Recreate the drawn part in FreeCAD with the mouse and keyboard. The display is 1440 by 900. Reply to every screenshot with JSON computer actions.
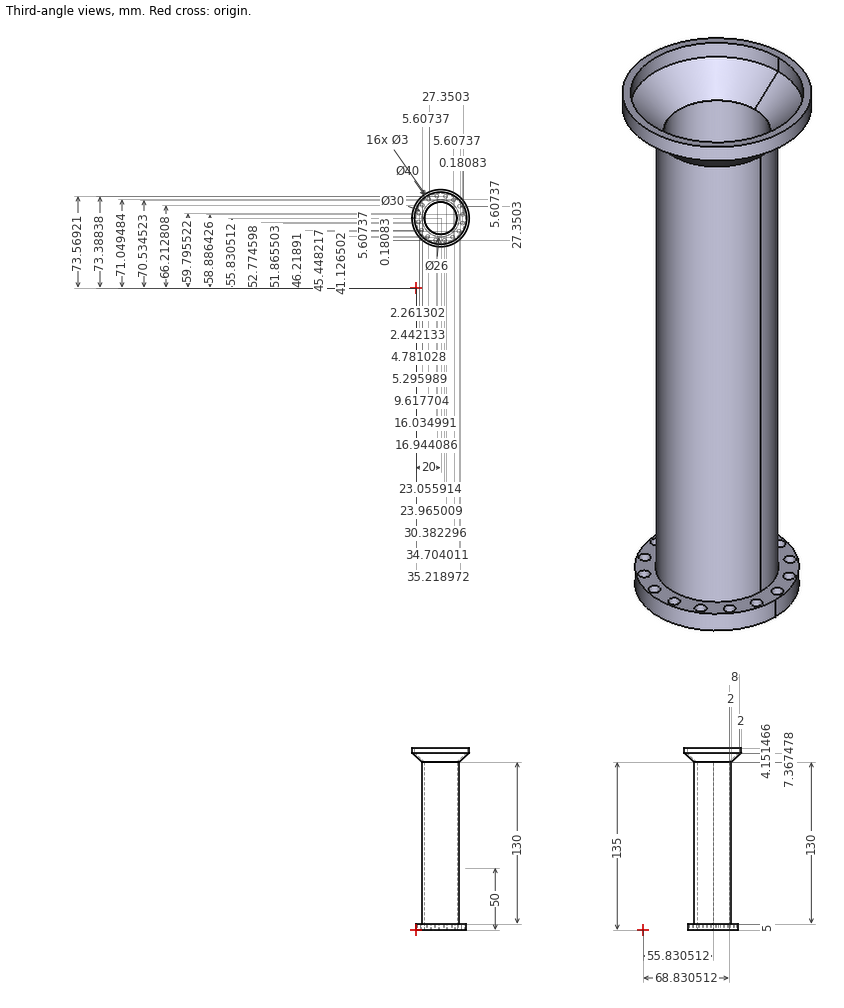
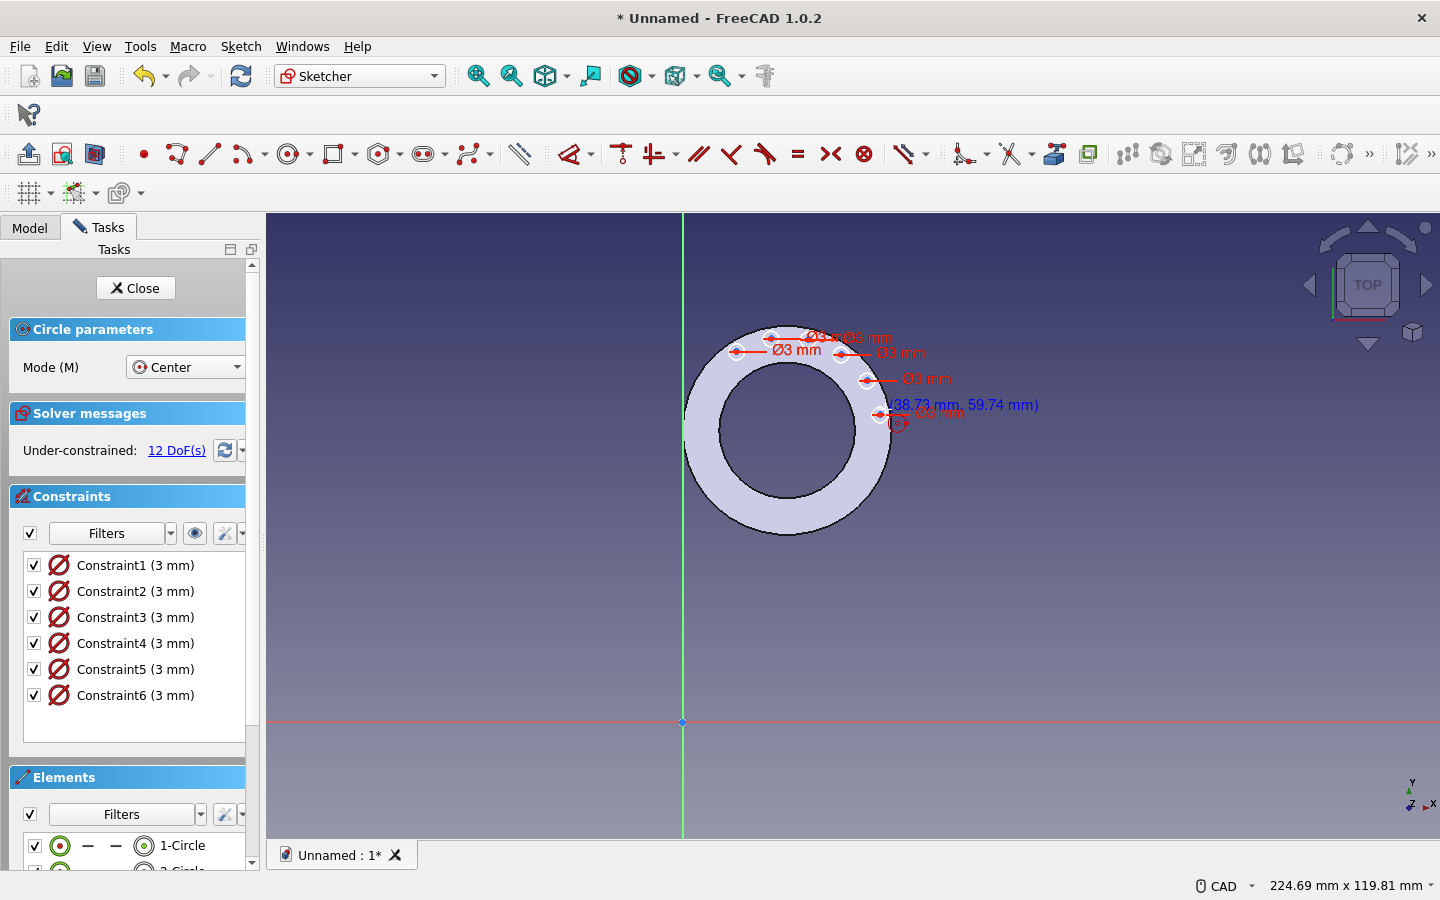
{"action": "scroll", "coordinate": [879, 451], "scroll_direction": "up", "scroll_amount": 6}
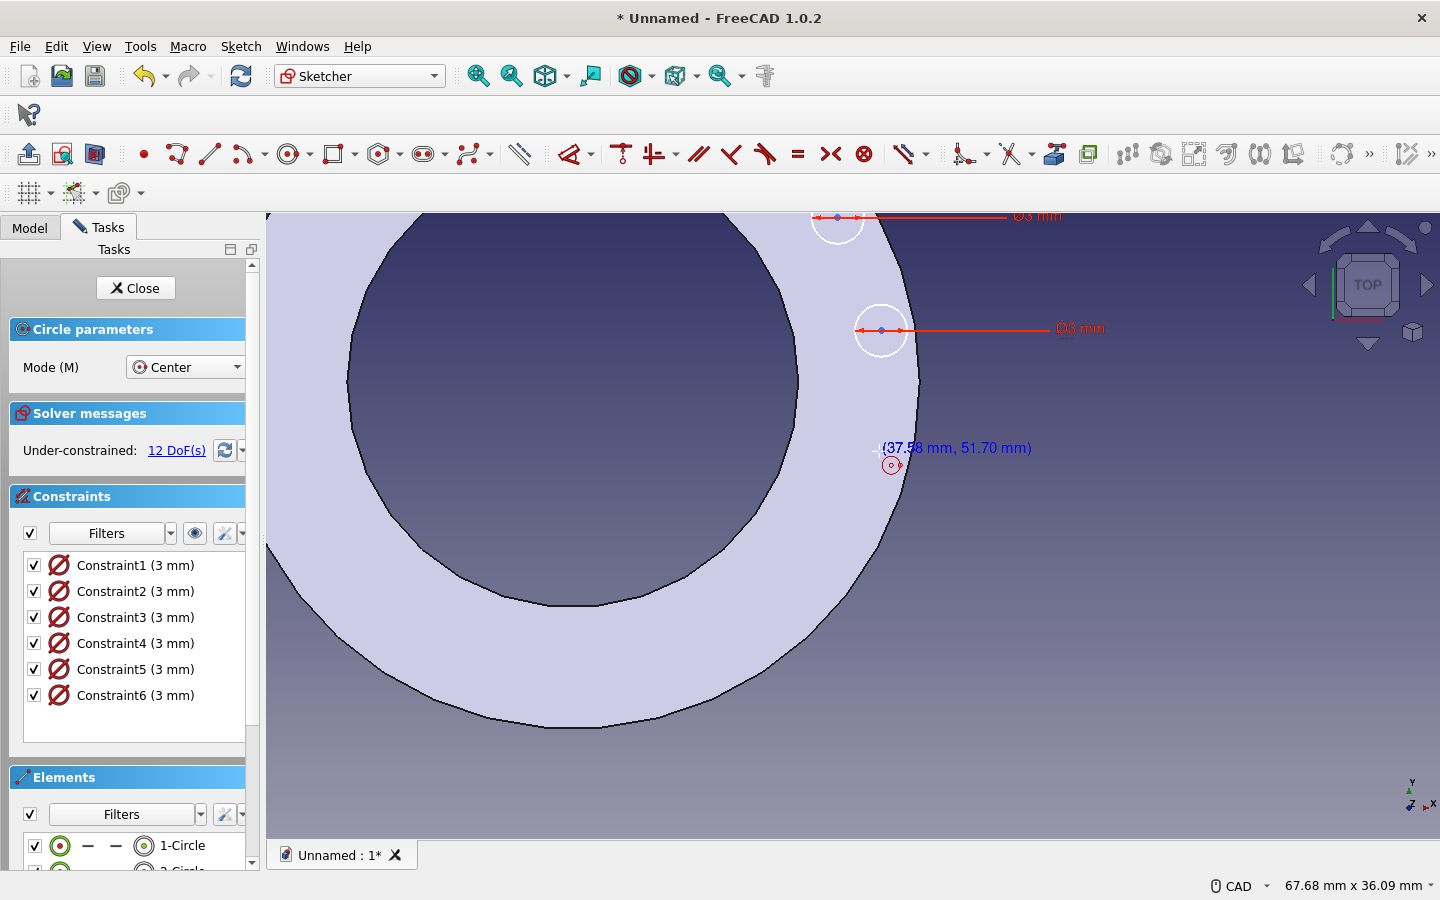
{"action": "scroll", "coordinate": [879, 451], "scroll_direction": "down", "scroll_amount": 6}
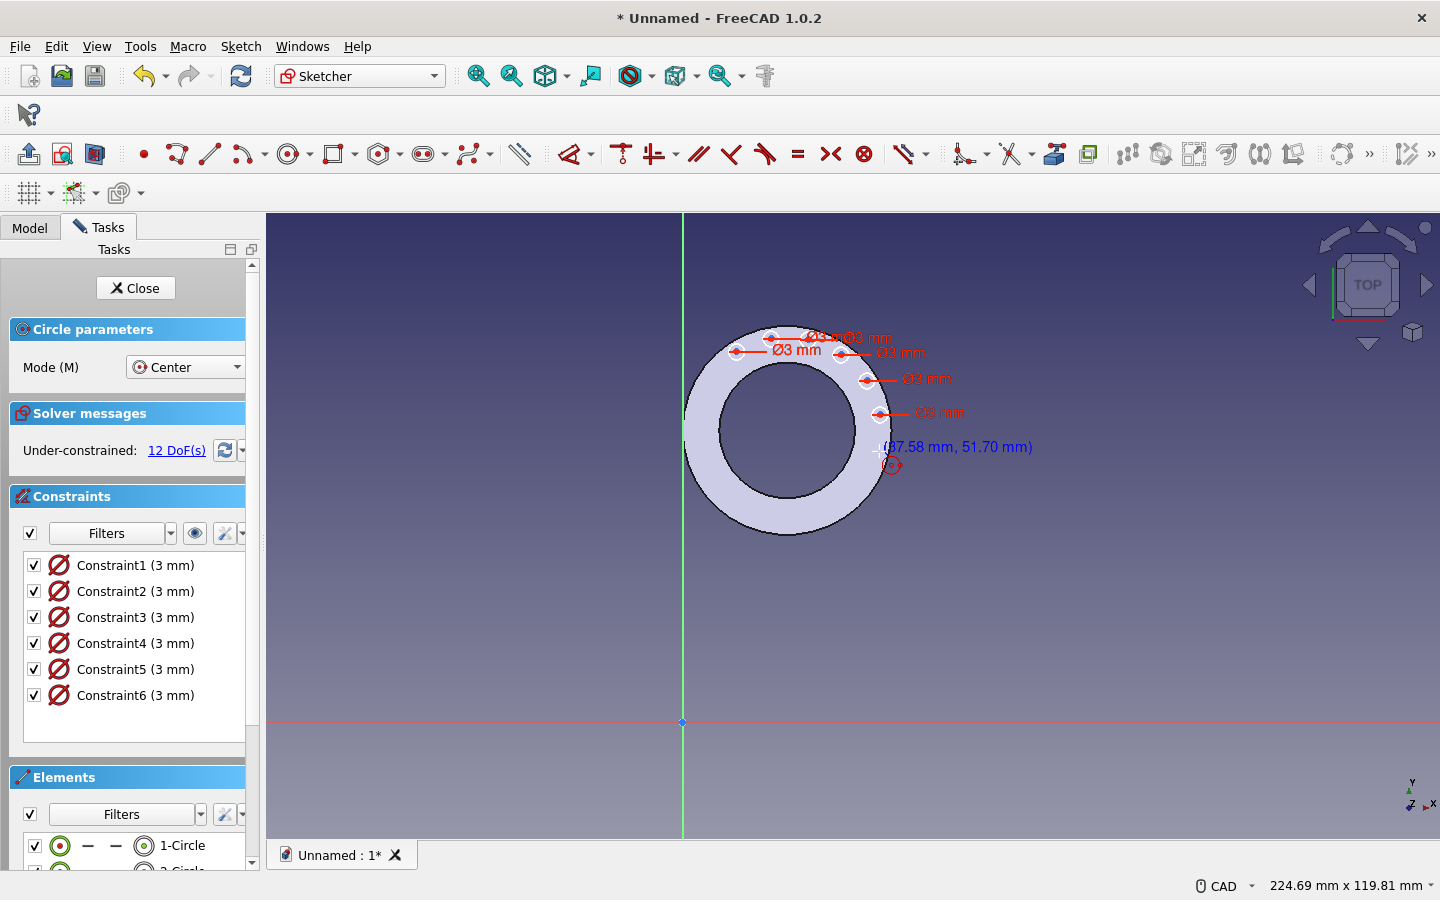
{"action": "left_click", "coordinate": [879, 451]}
{"action": "mouse_move", "coordinate": [884, 446]}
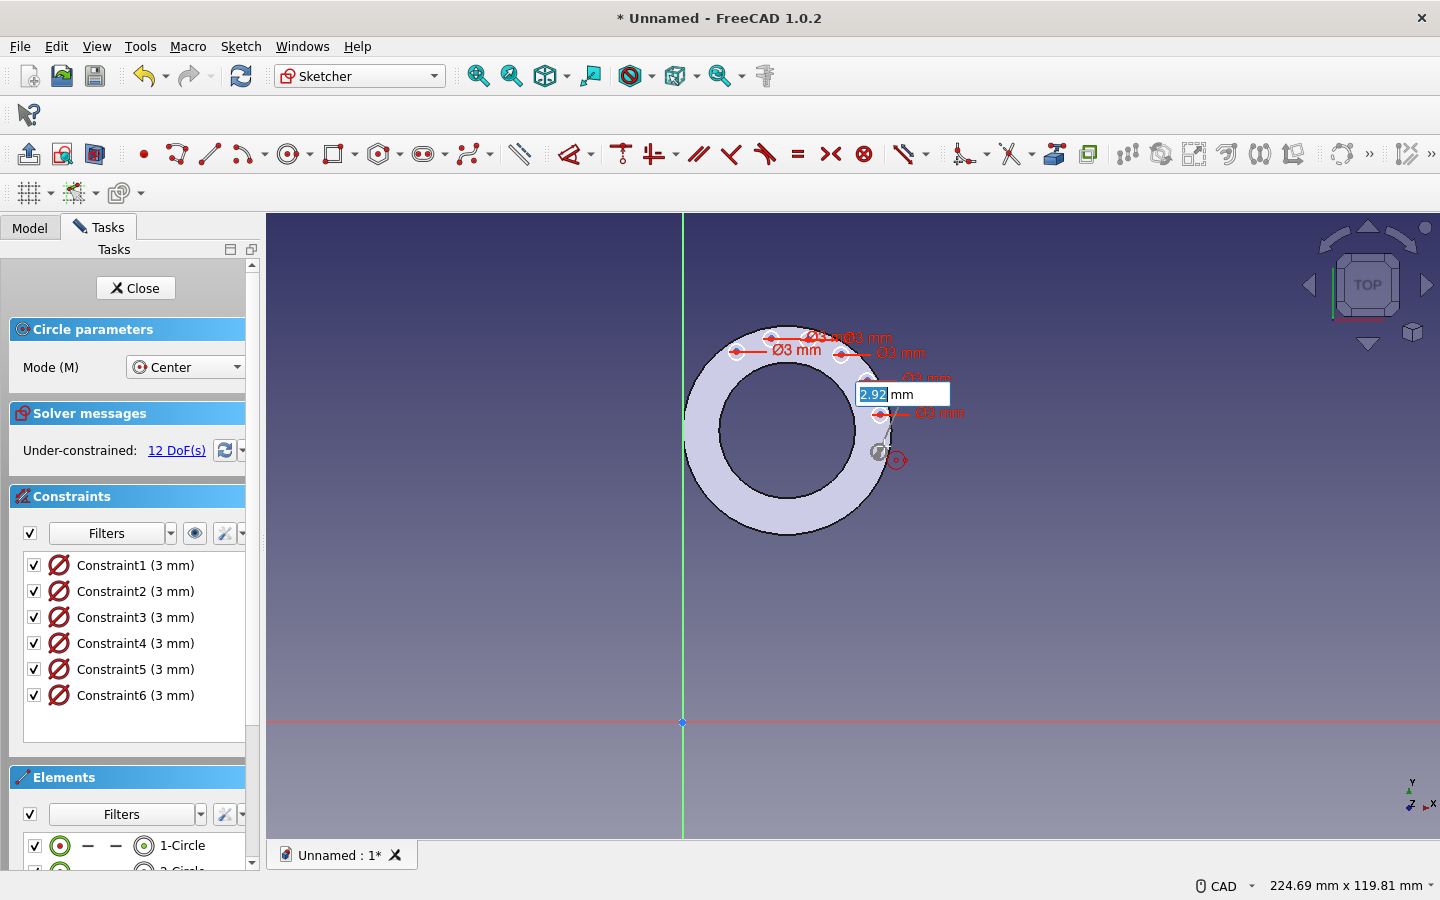
{"action": "type", "text": "3"}
{"action": "key", "text": "Return"}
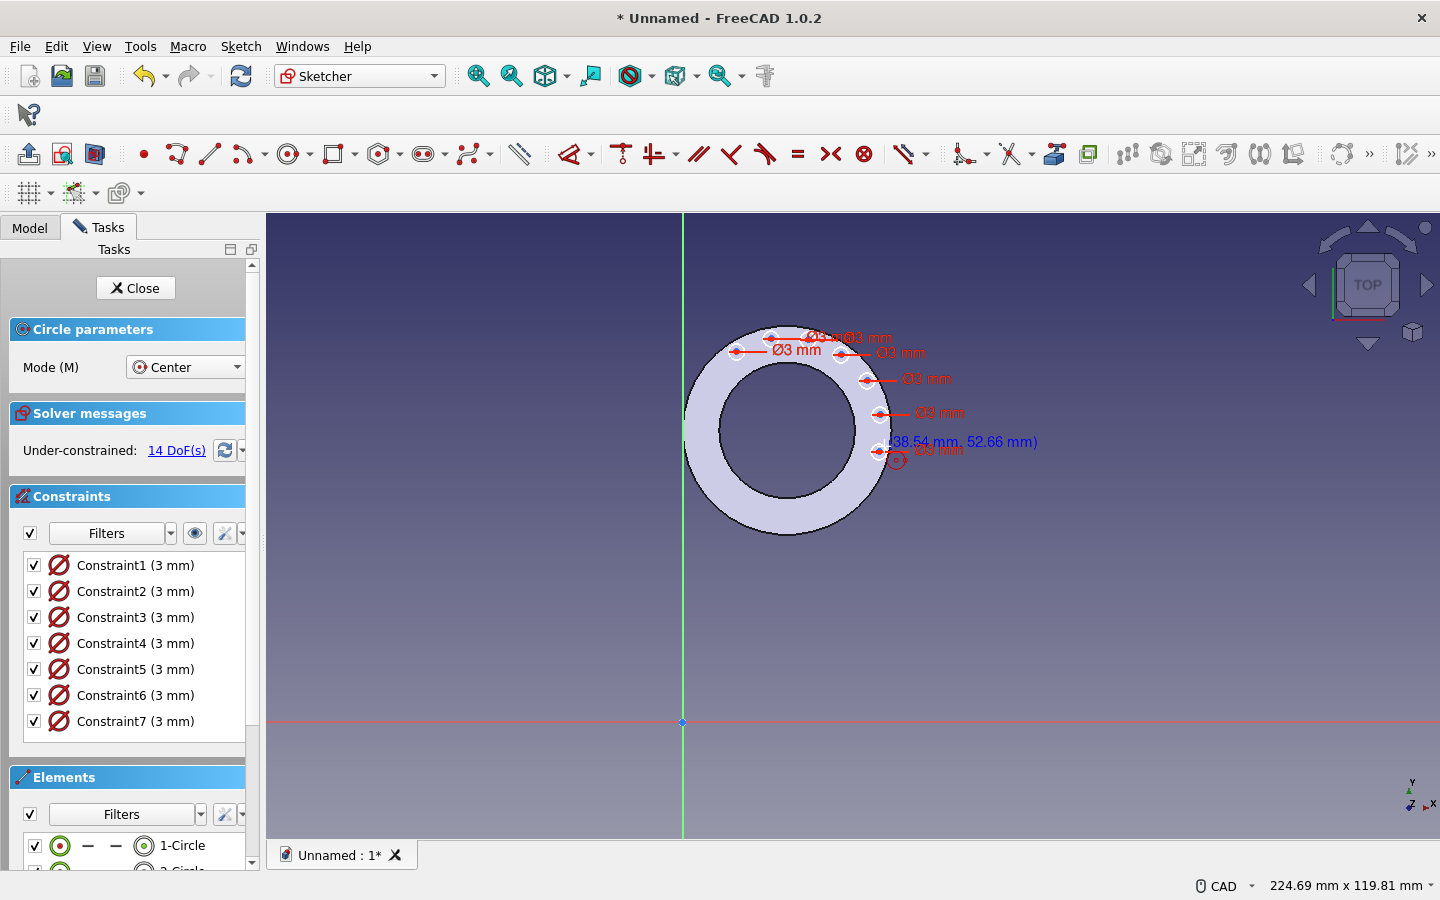
{"action": "scroll", "coordinate": [864, 485], "scroll_direction": "up", "scroll_amount": 6}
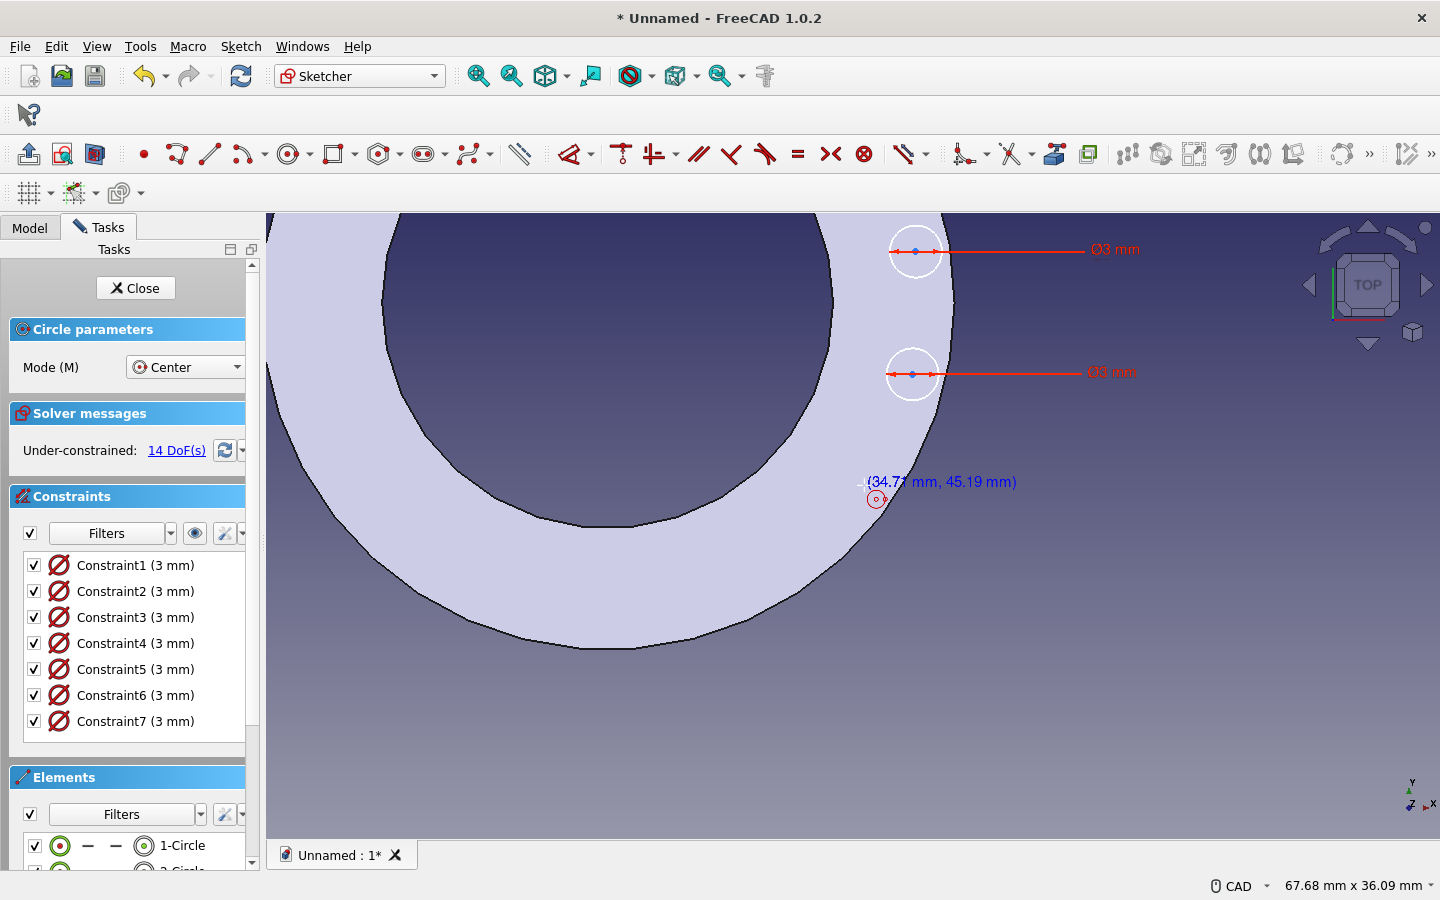
{"action": "scroll", "coordinate": [864, 485], "scroll_direction": "down", "scroll_amount": 6}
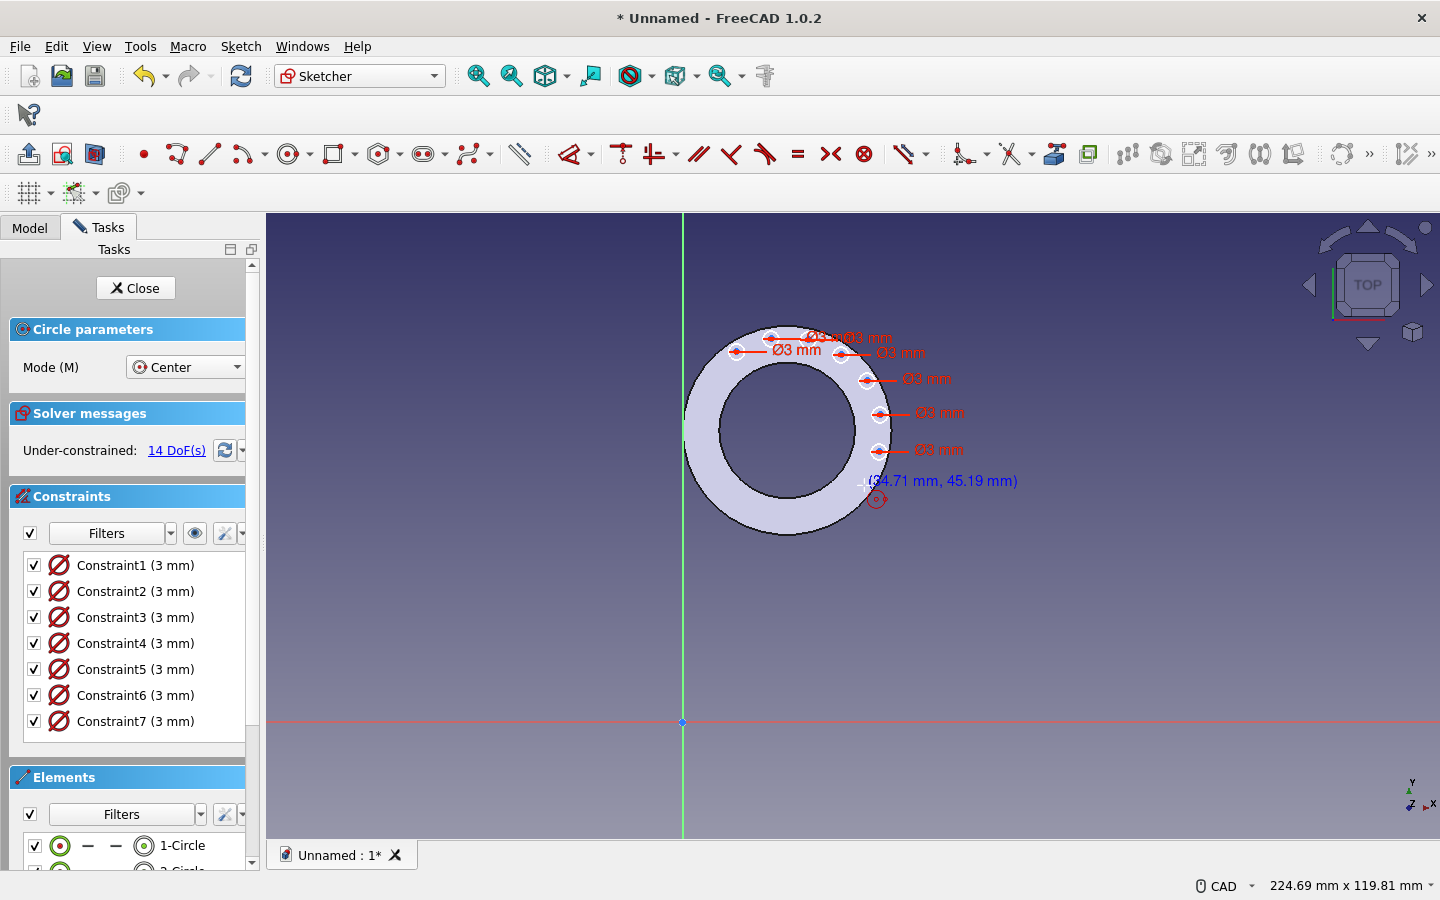
{"action": "left_click", "coordinate": [864, 485]}
{"action": "mouse_move", "coordinate": [870, 479]}